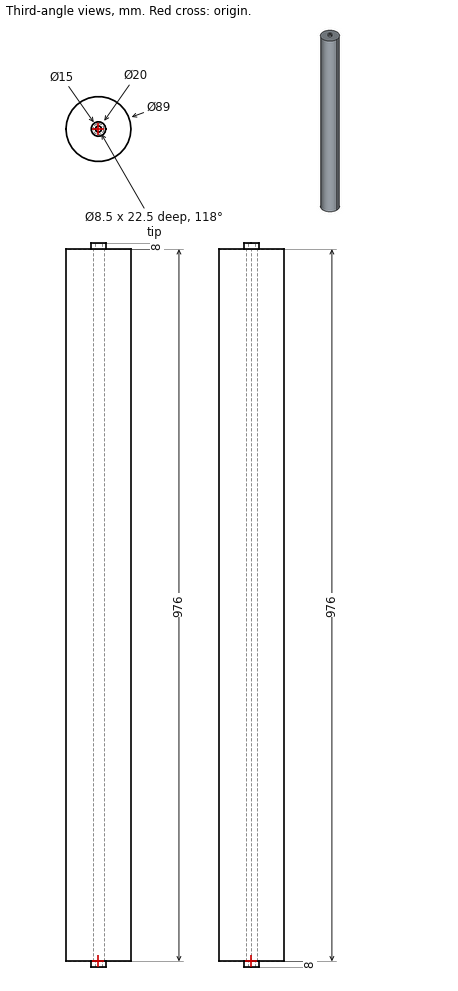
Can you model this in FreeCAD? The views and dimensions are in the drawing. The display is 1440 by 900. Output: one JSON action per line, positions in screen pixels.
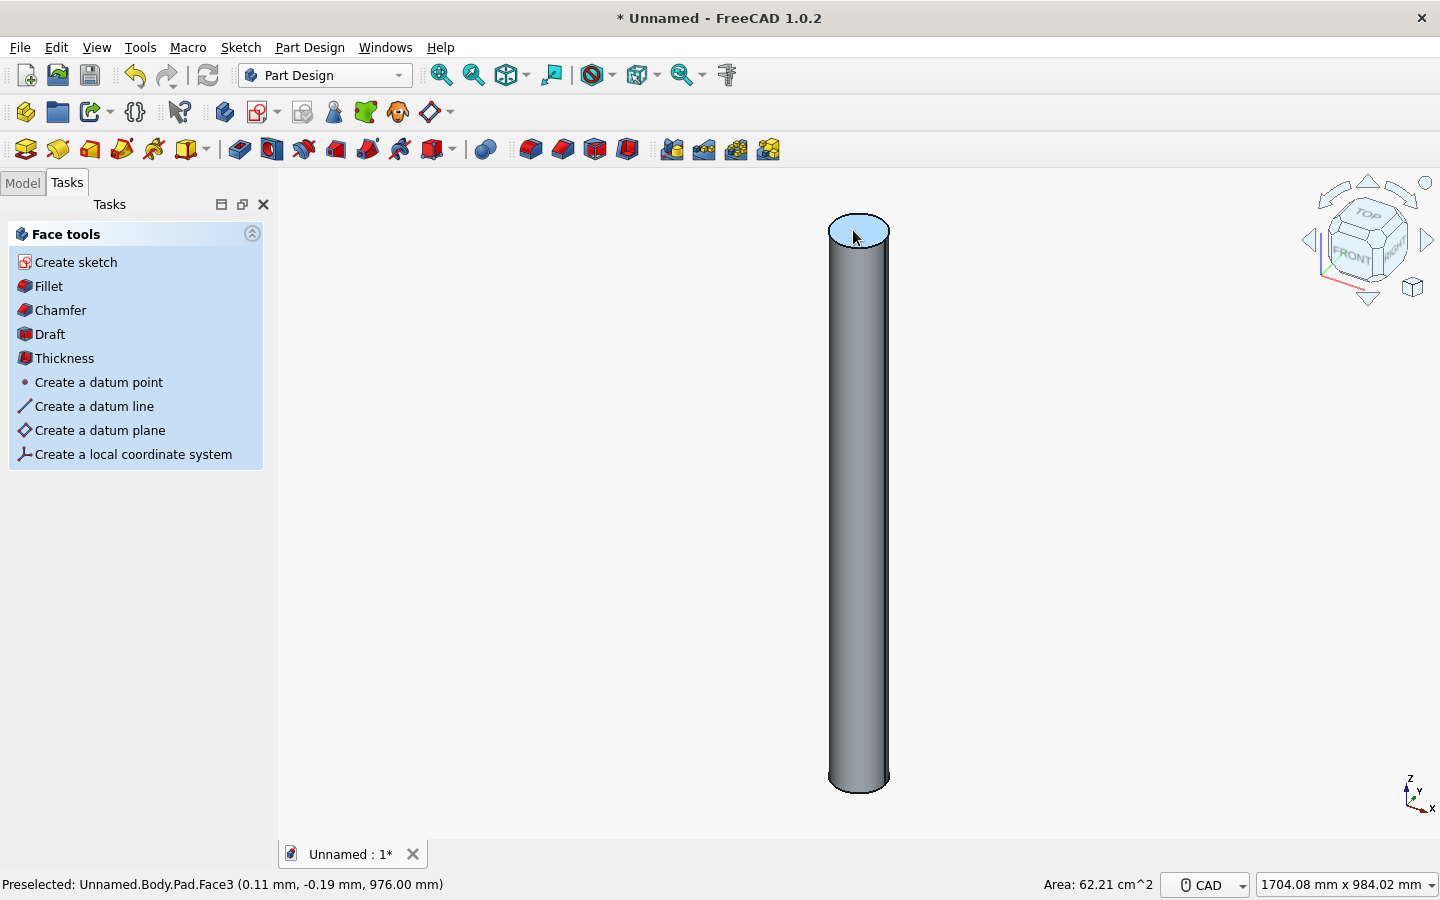
{"action": "left_click", "coordinate": [258, 112]}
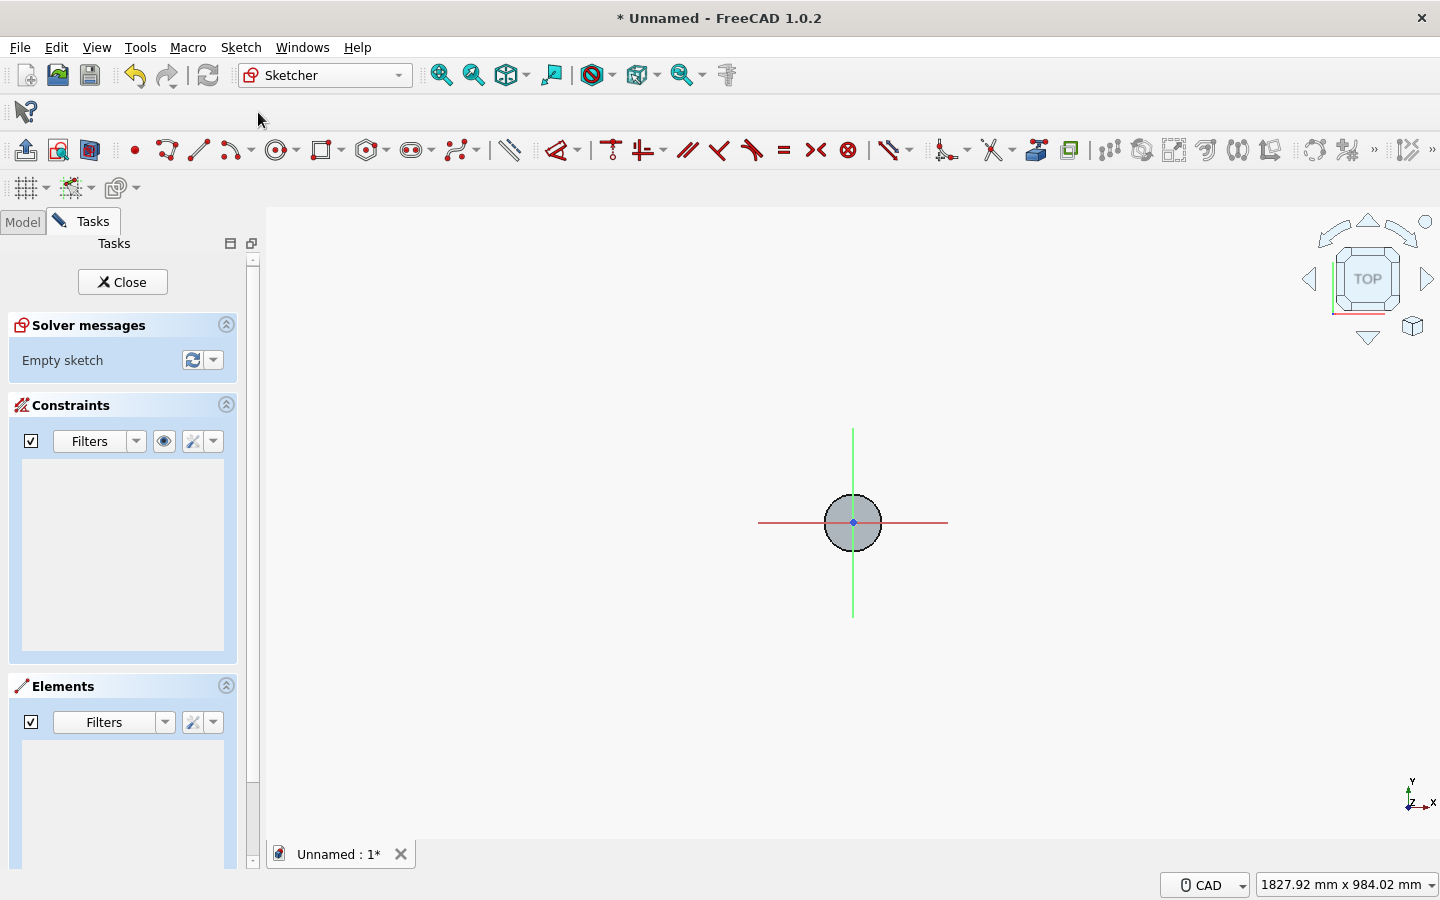
{"action": "scroll", "coordinate": [857, 523], "scroll_direction": "up", "scroll_amount": 15}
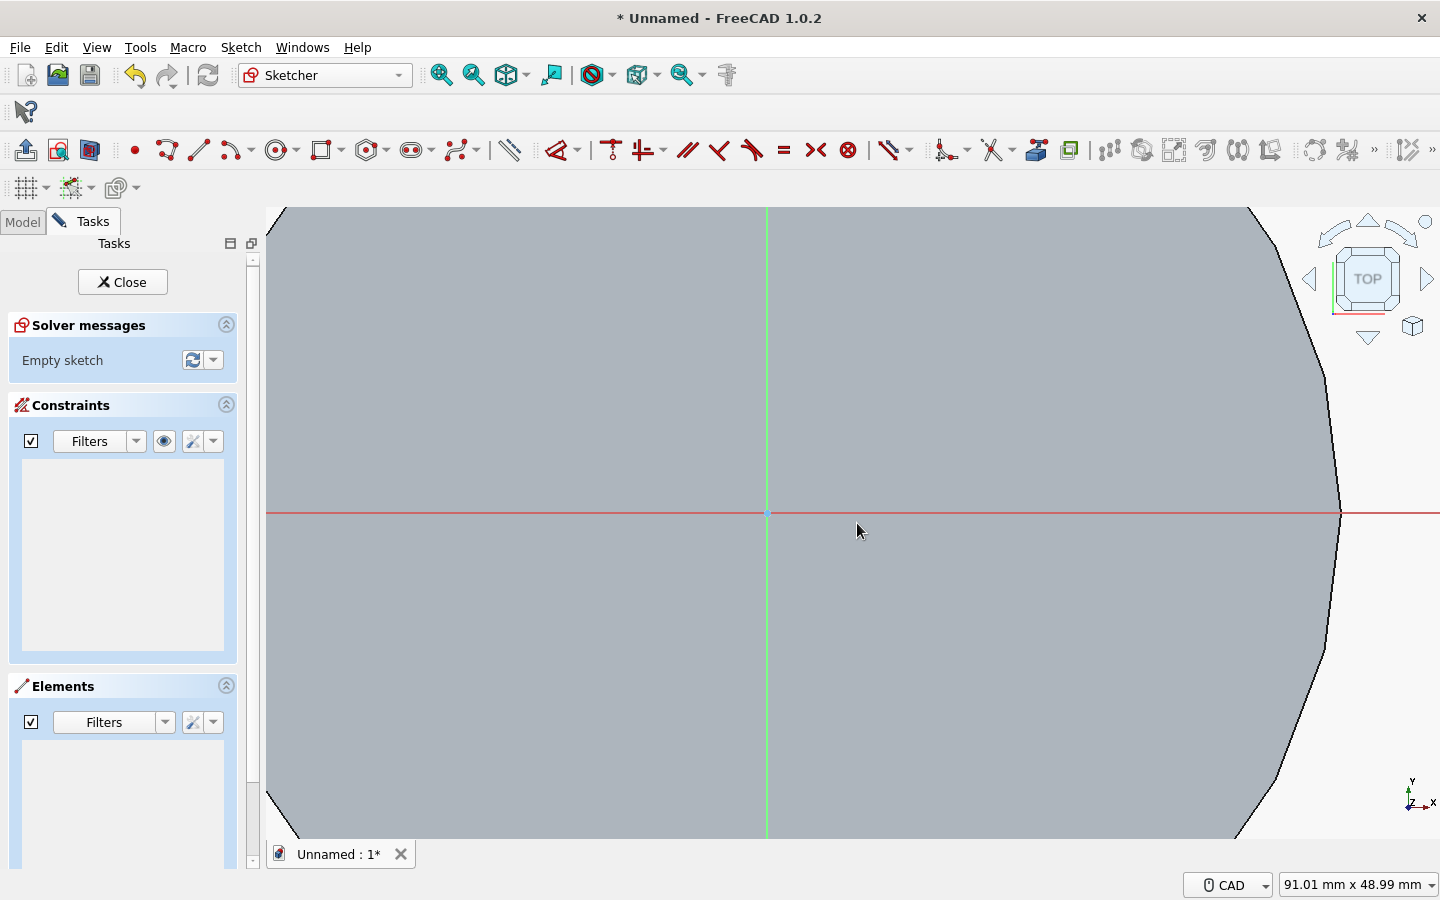
{"action": "scroll", "coordinate": [732, 494], "scroll_direction": "up", "scroll_amount": 2}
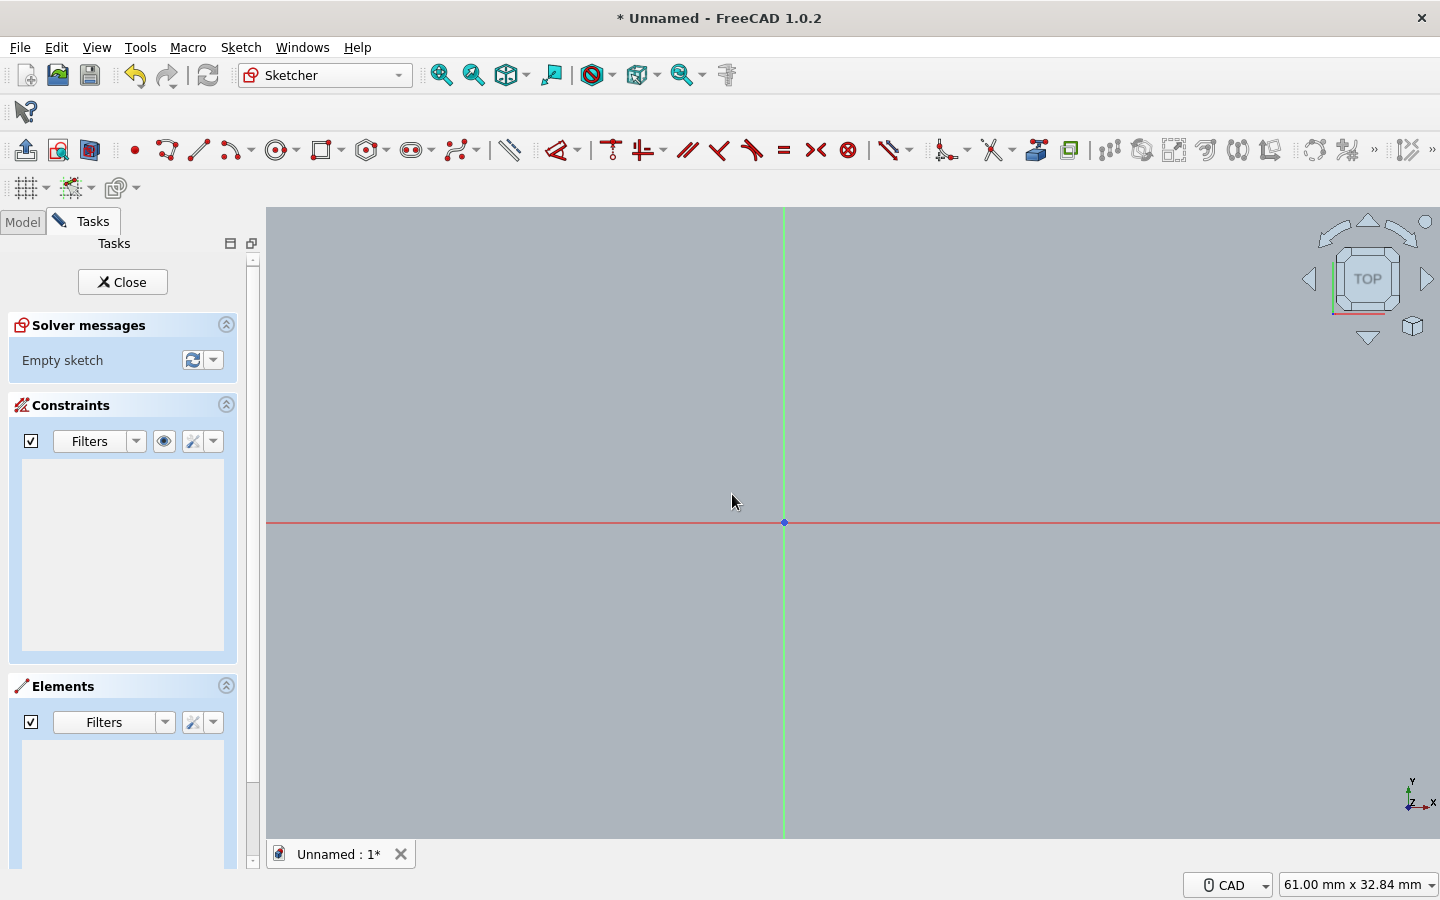
{"action": "left_click", "coordinate": [276, 150]}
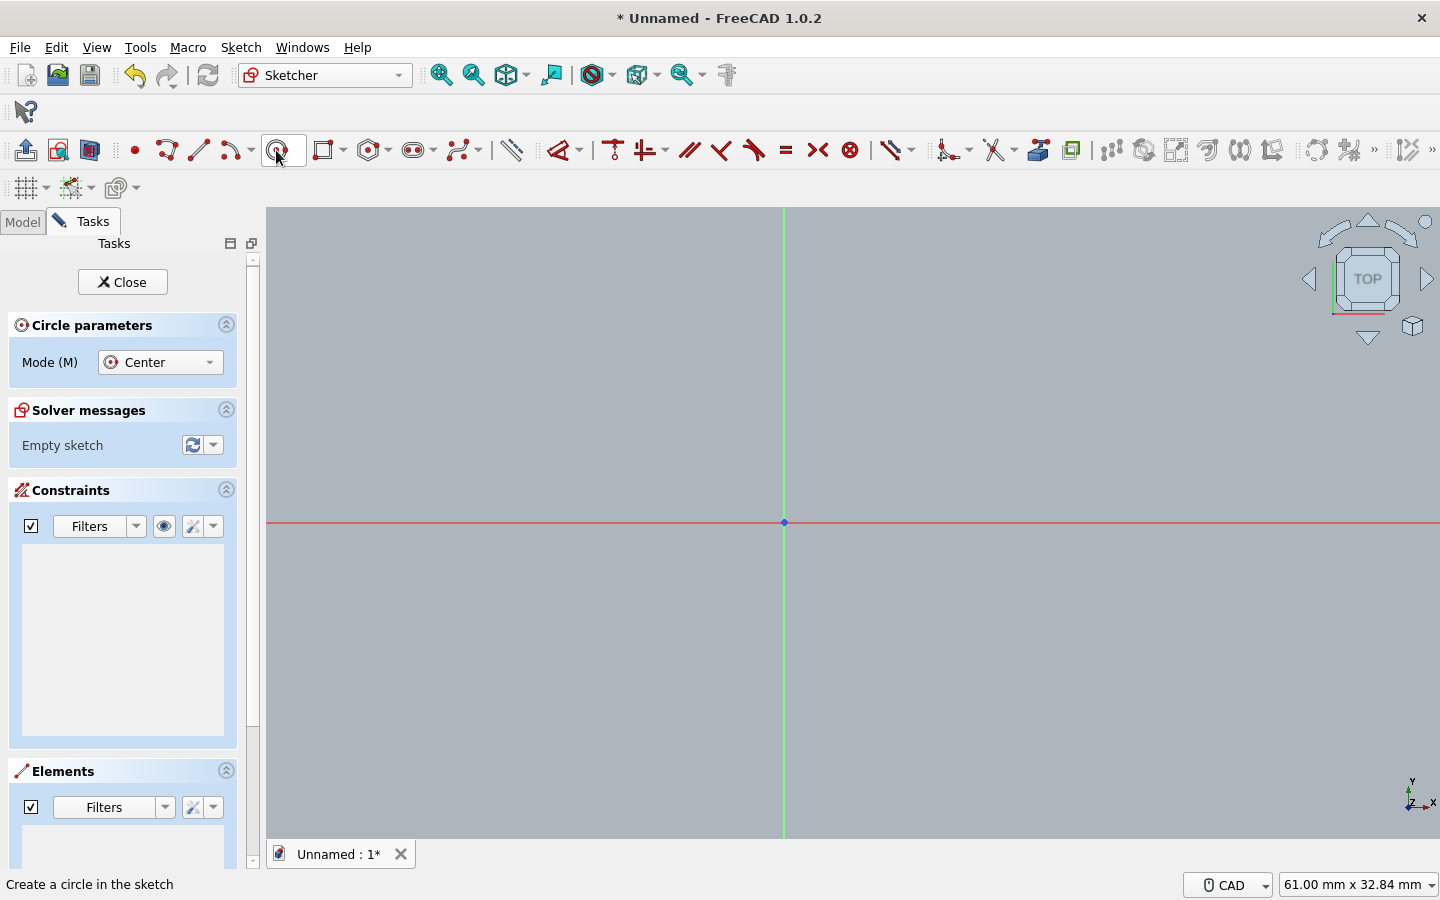
{"action": "left_click", "coordinate": [784, 523]}
{"action": "left_click", "coordinate": [920, 387]}
{"action": "key", "text": "Escape"}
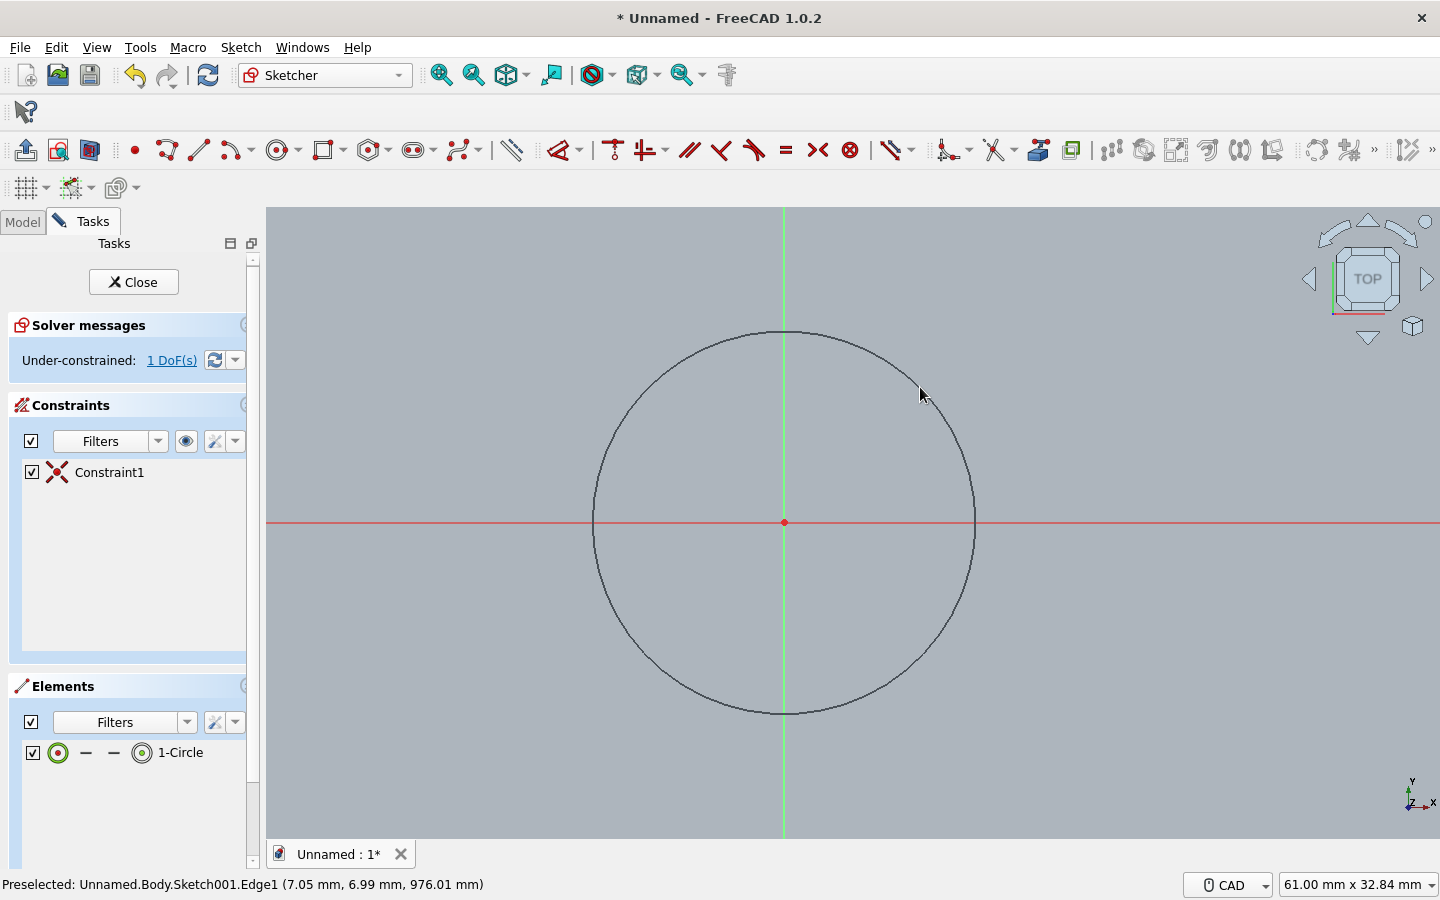
{"action": "left_click", "coordinate": [558, 150]}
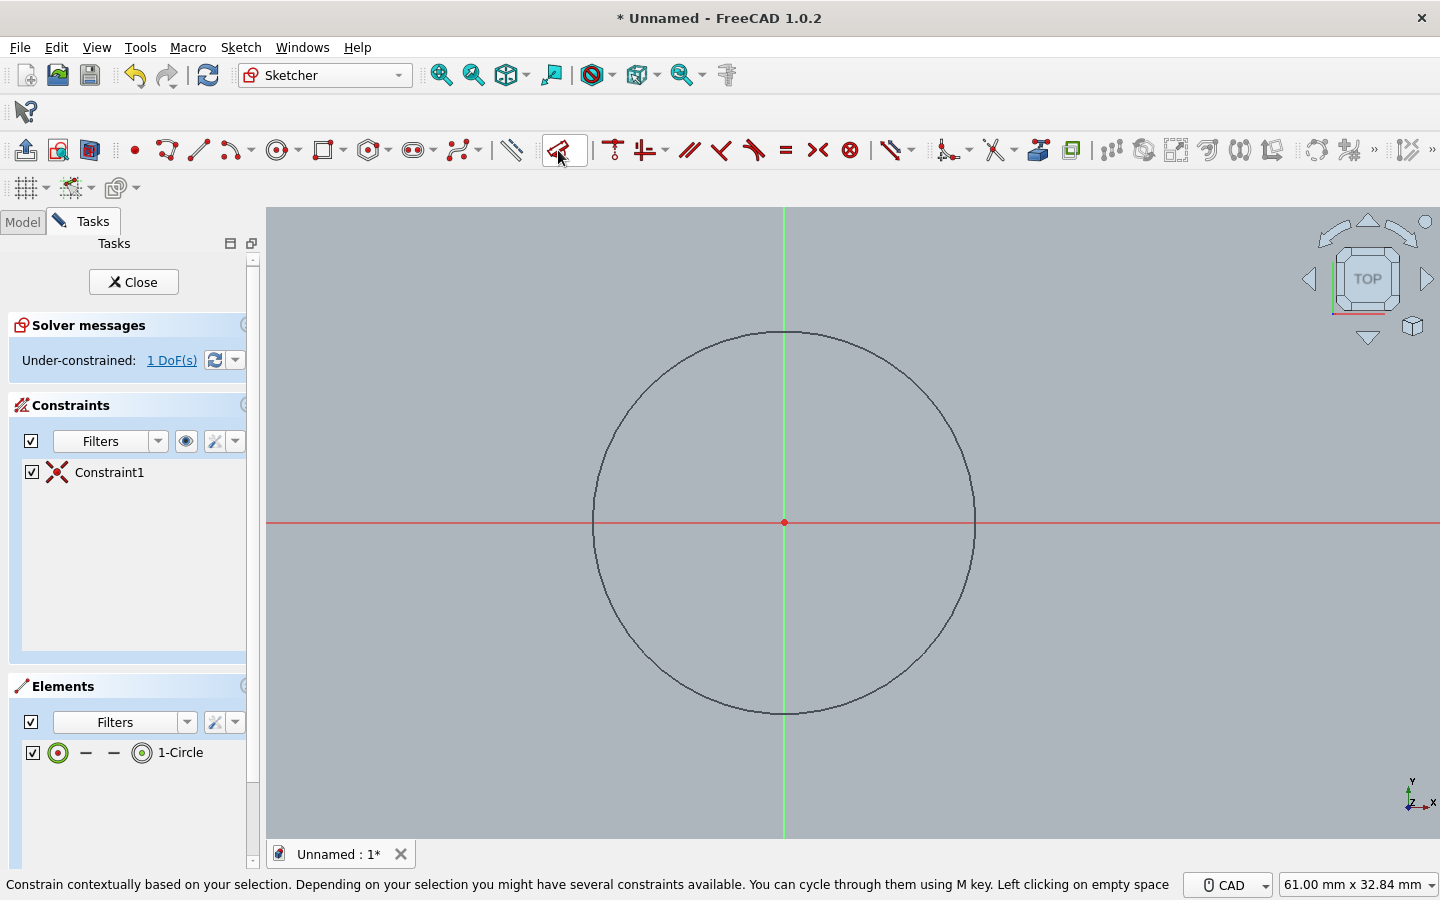
{"action": "left_click", "coordinate": [919, 387]}
{"action": "left_click", "coordinate": [942, 364]}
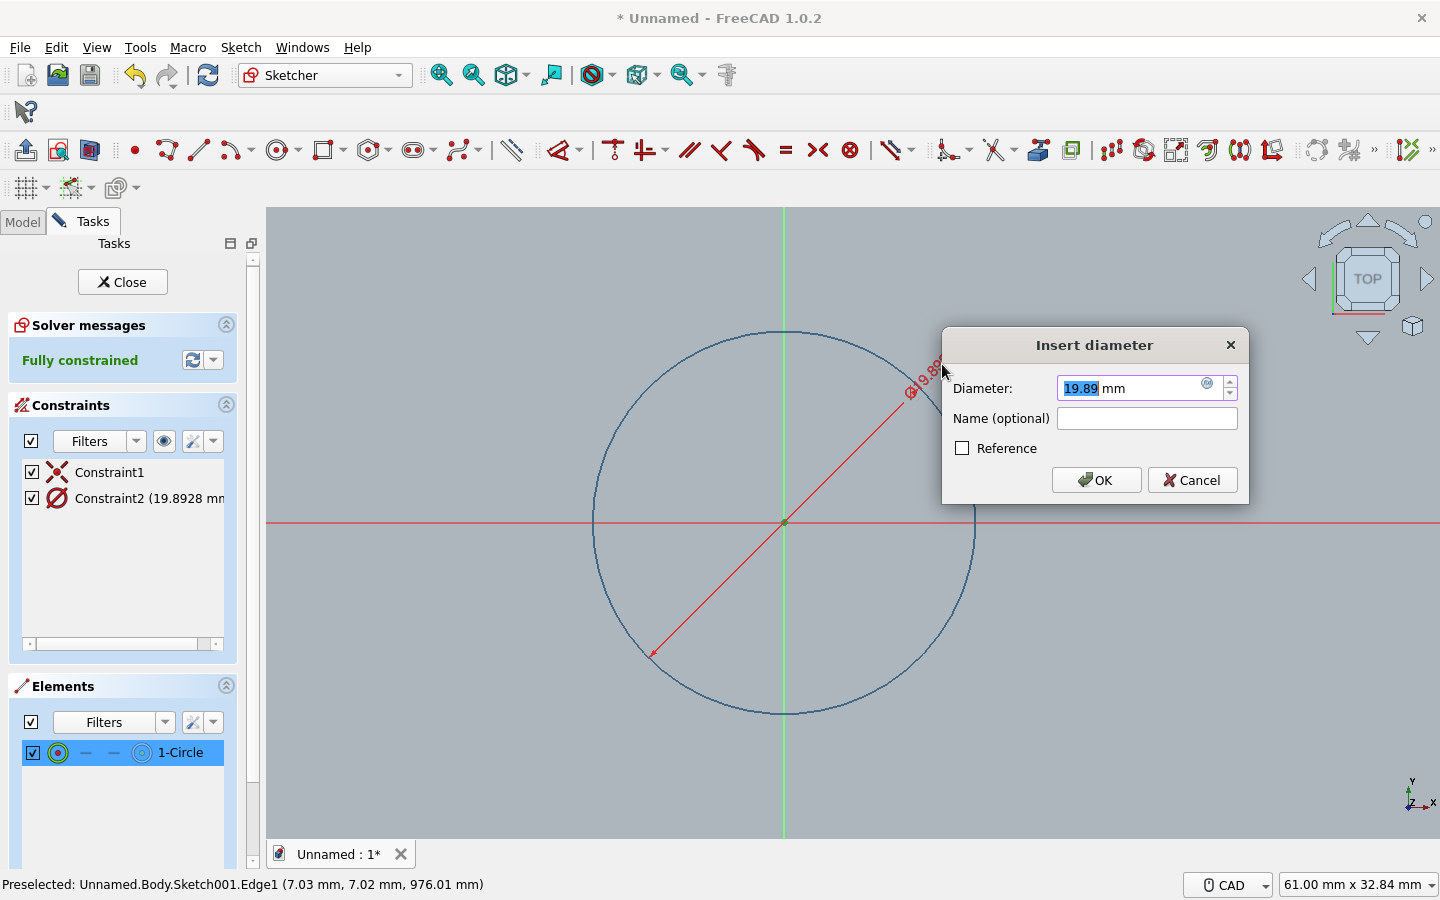
{"action": "type", "text": "20"}
{"action": "key", "text": "Return"}
{"action": "key", "text": "Escape"}